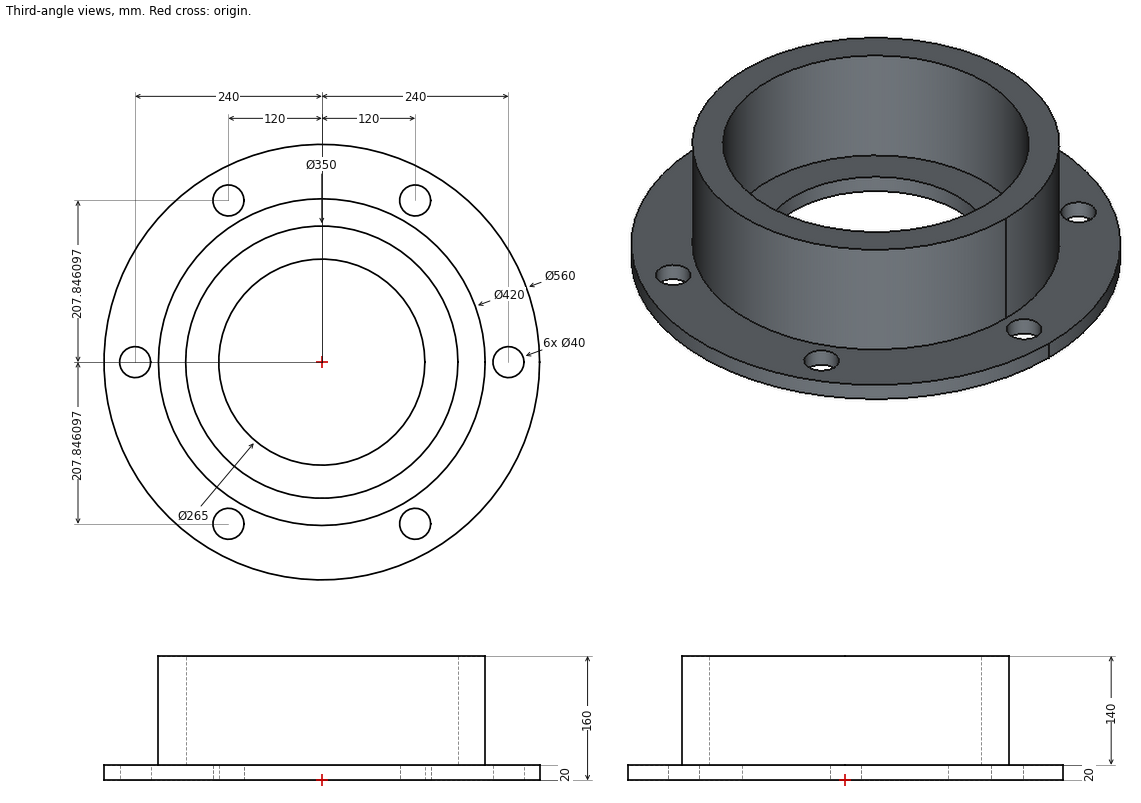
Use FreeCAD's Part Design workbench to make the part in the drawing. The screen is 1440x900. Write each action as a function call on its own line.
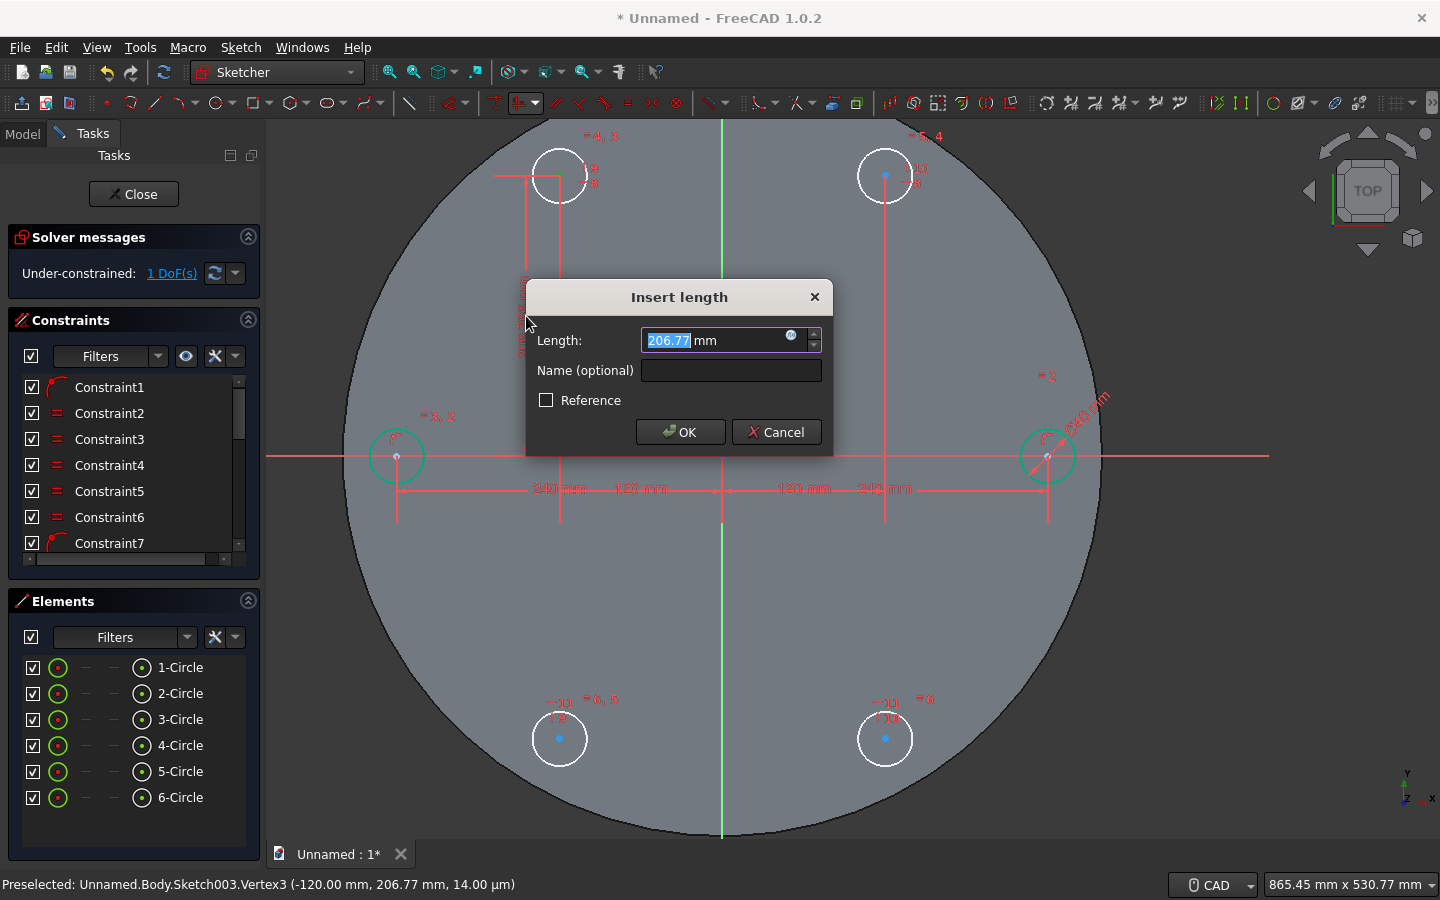
text(207.846097)
key(Return)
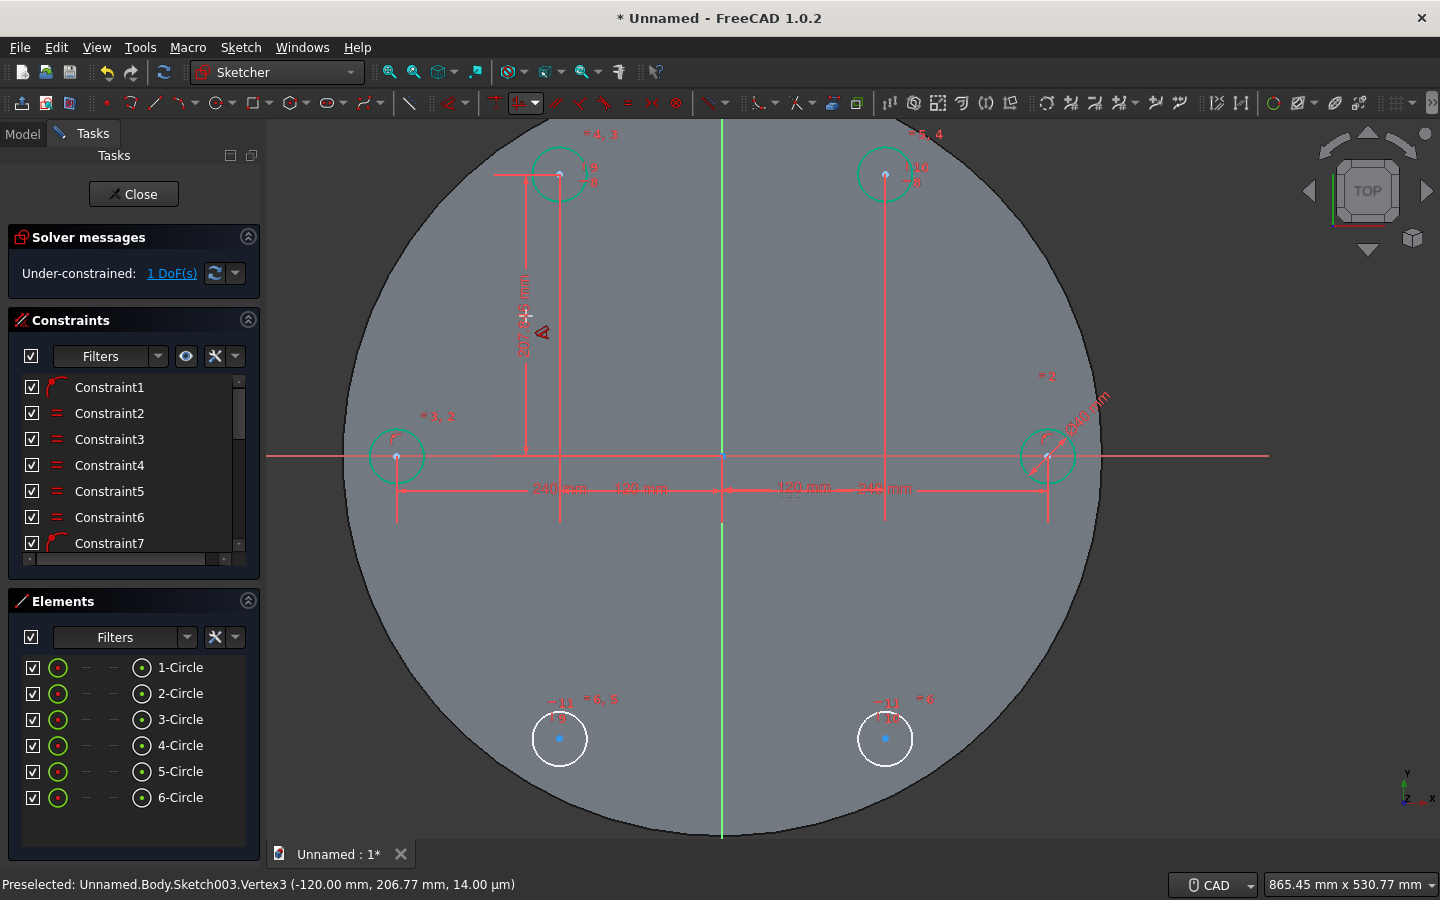
click(560, 739)
click(526, 598)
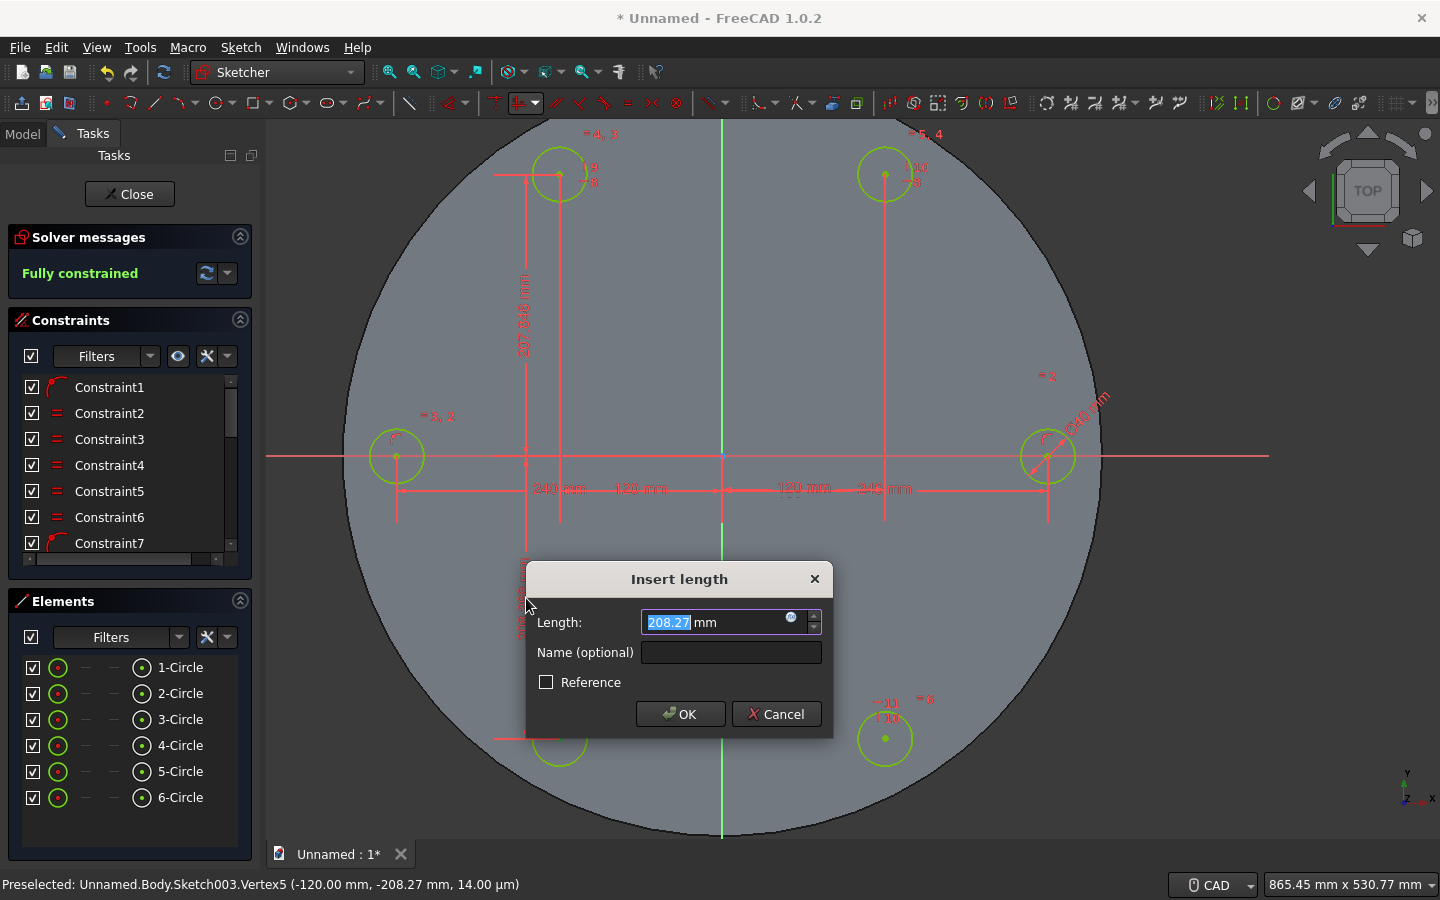
text(207.846097)
key(Return)
key(Escape)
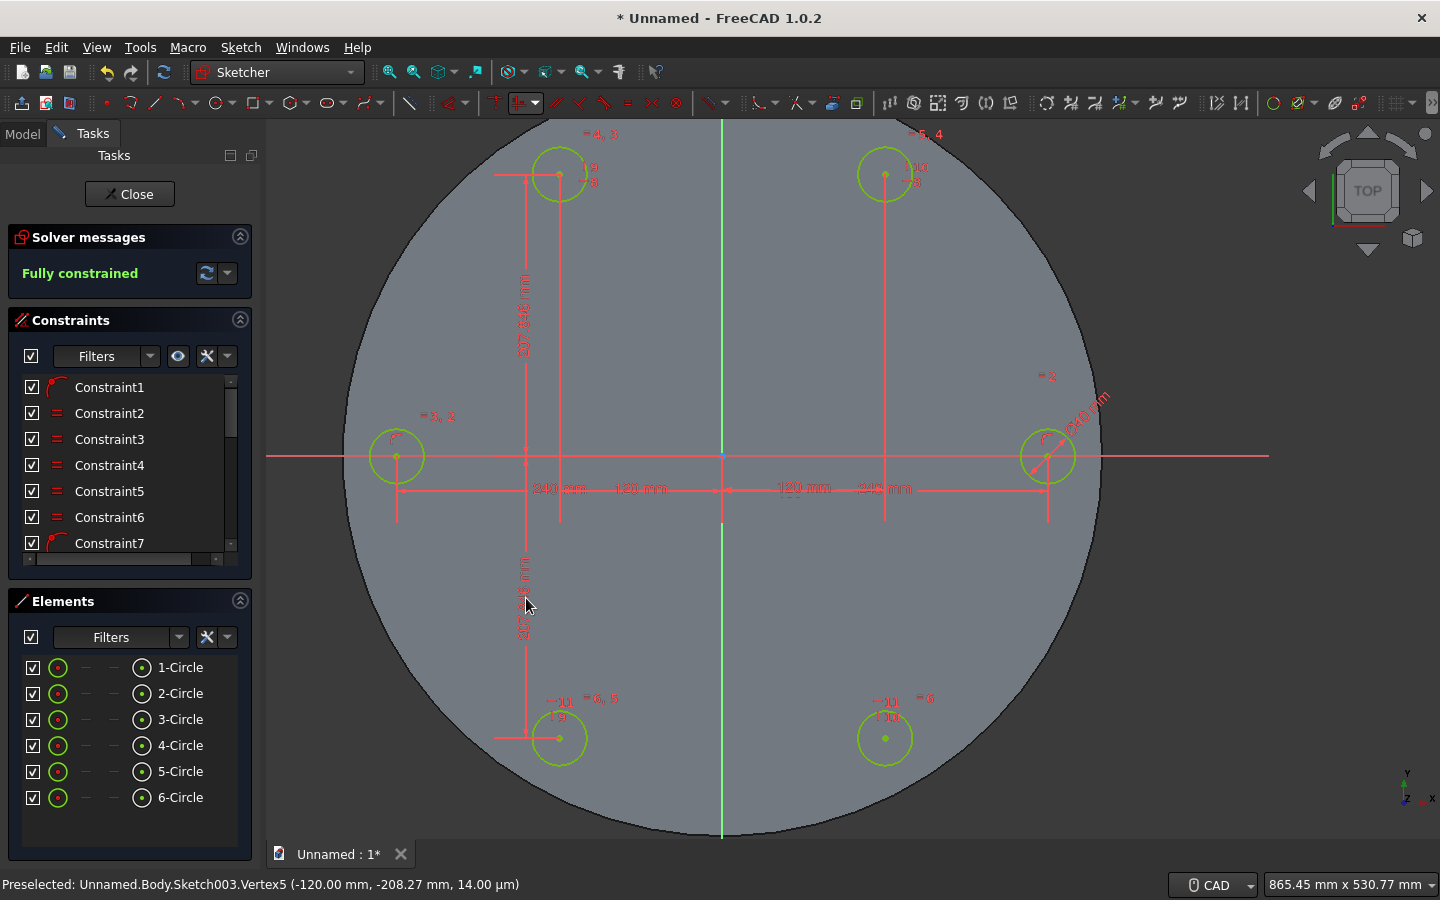
click(130, 194)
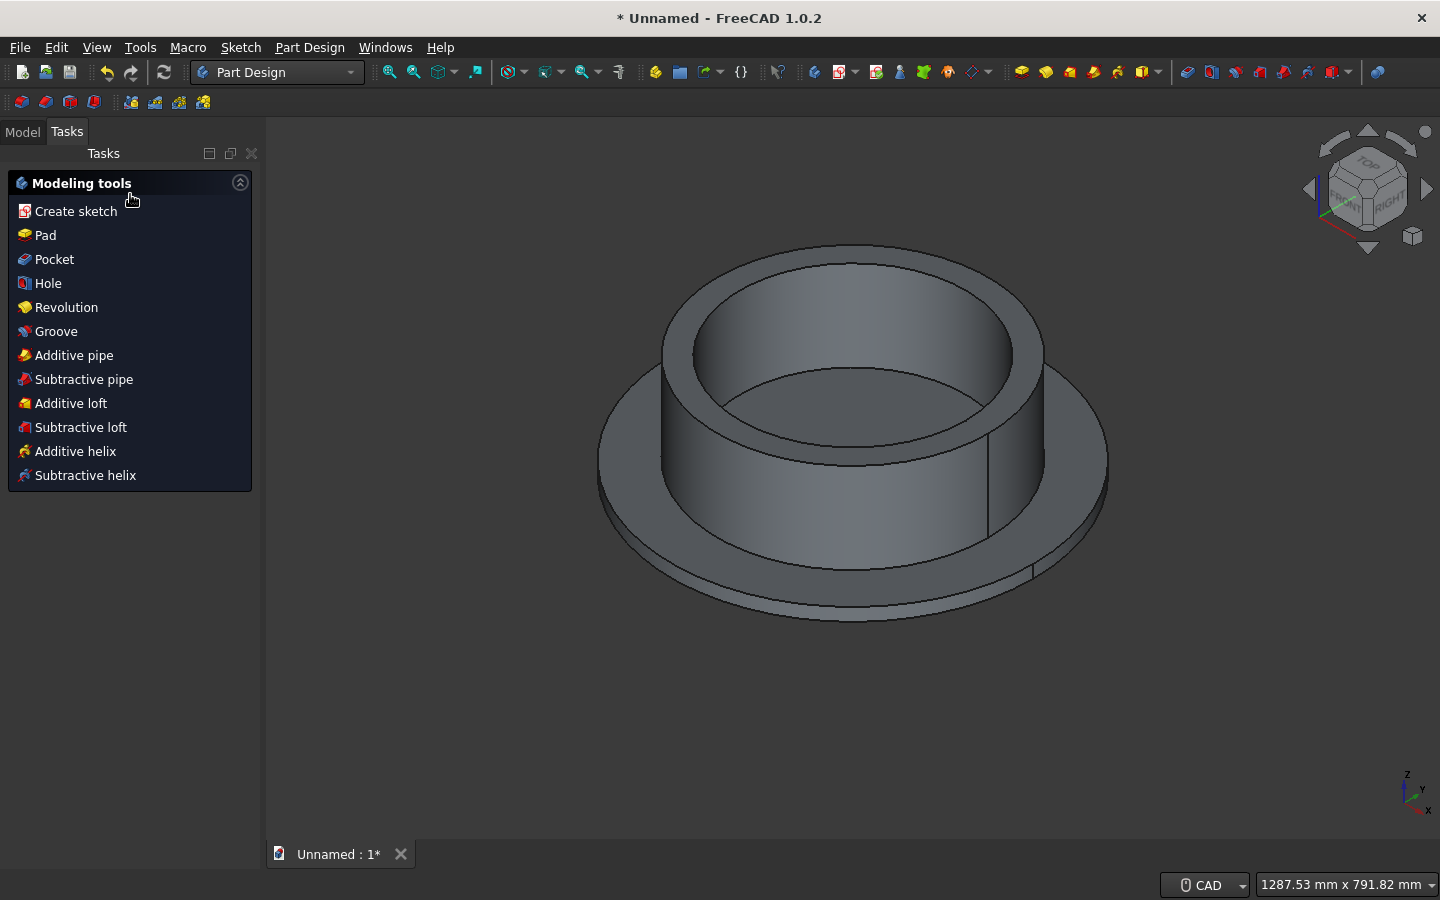
click(1188, 72)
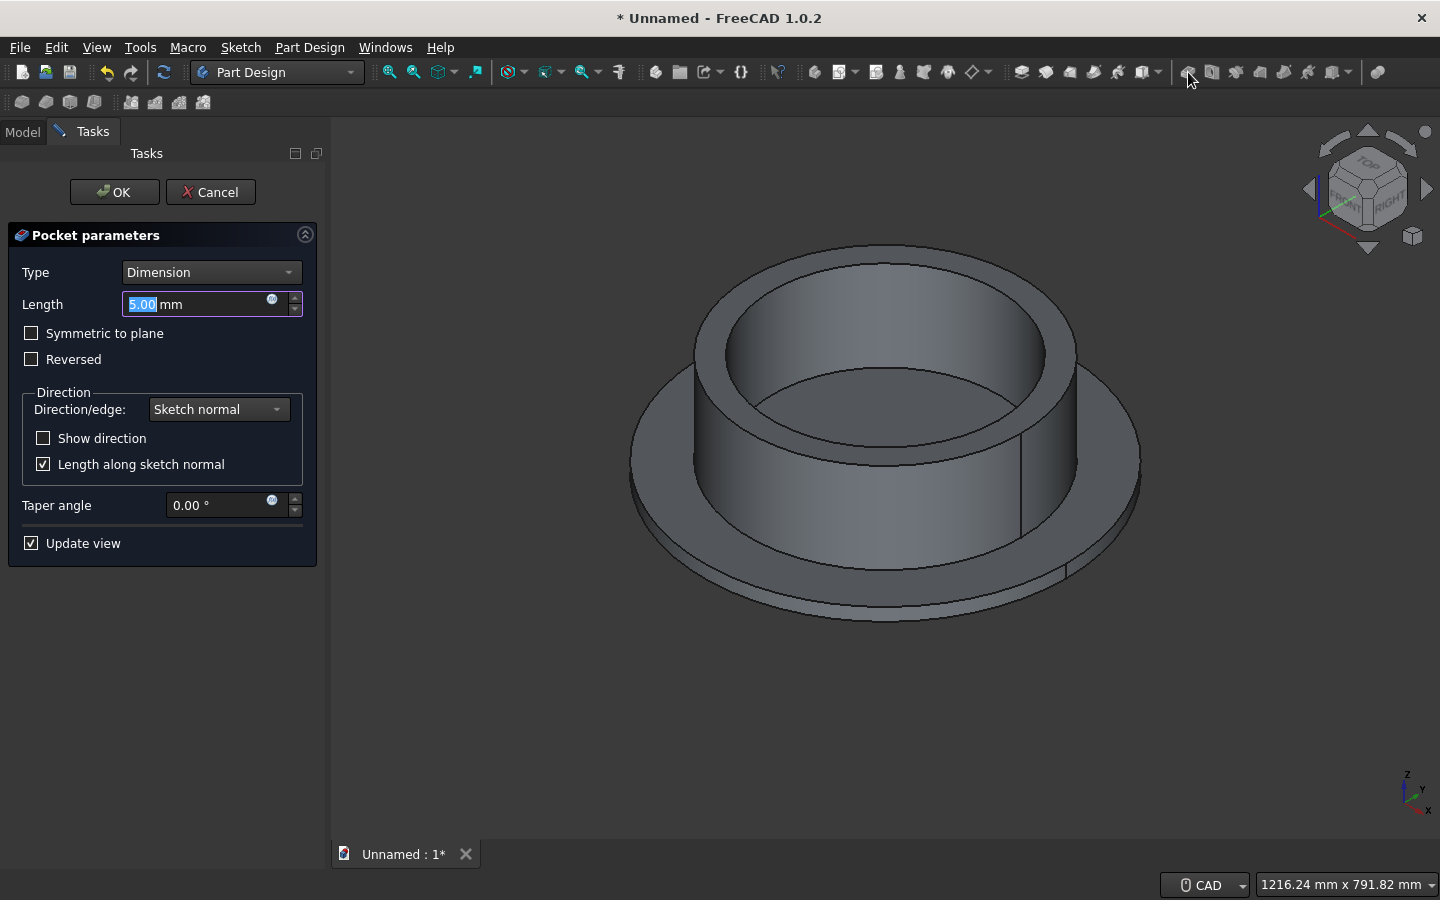
text(20)
key(Tab)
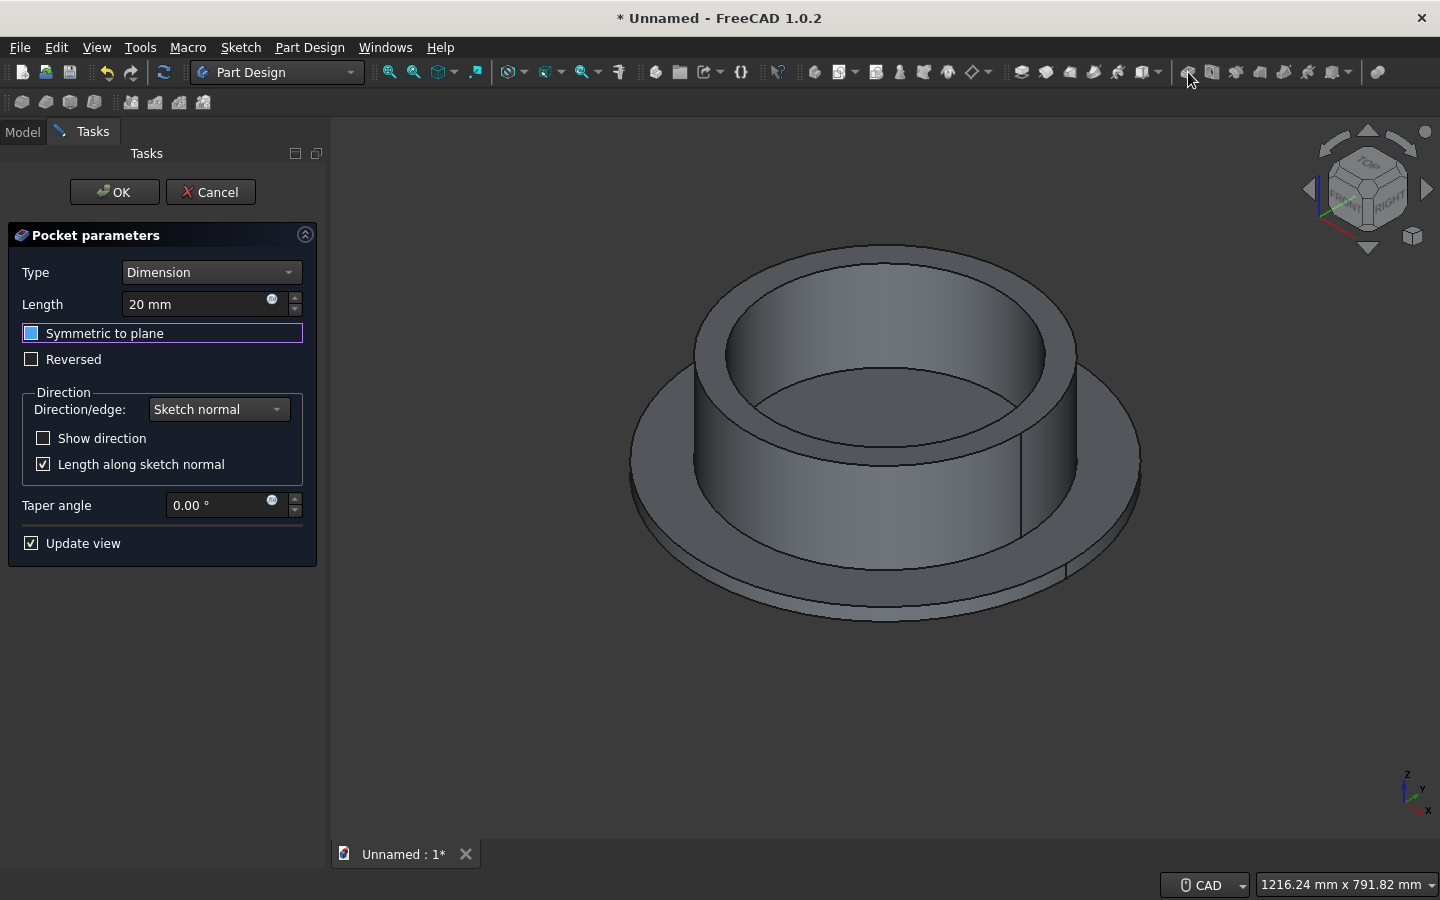
click(30, 359)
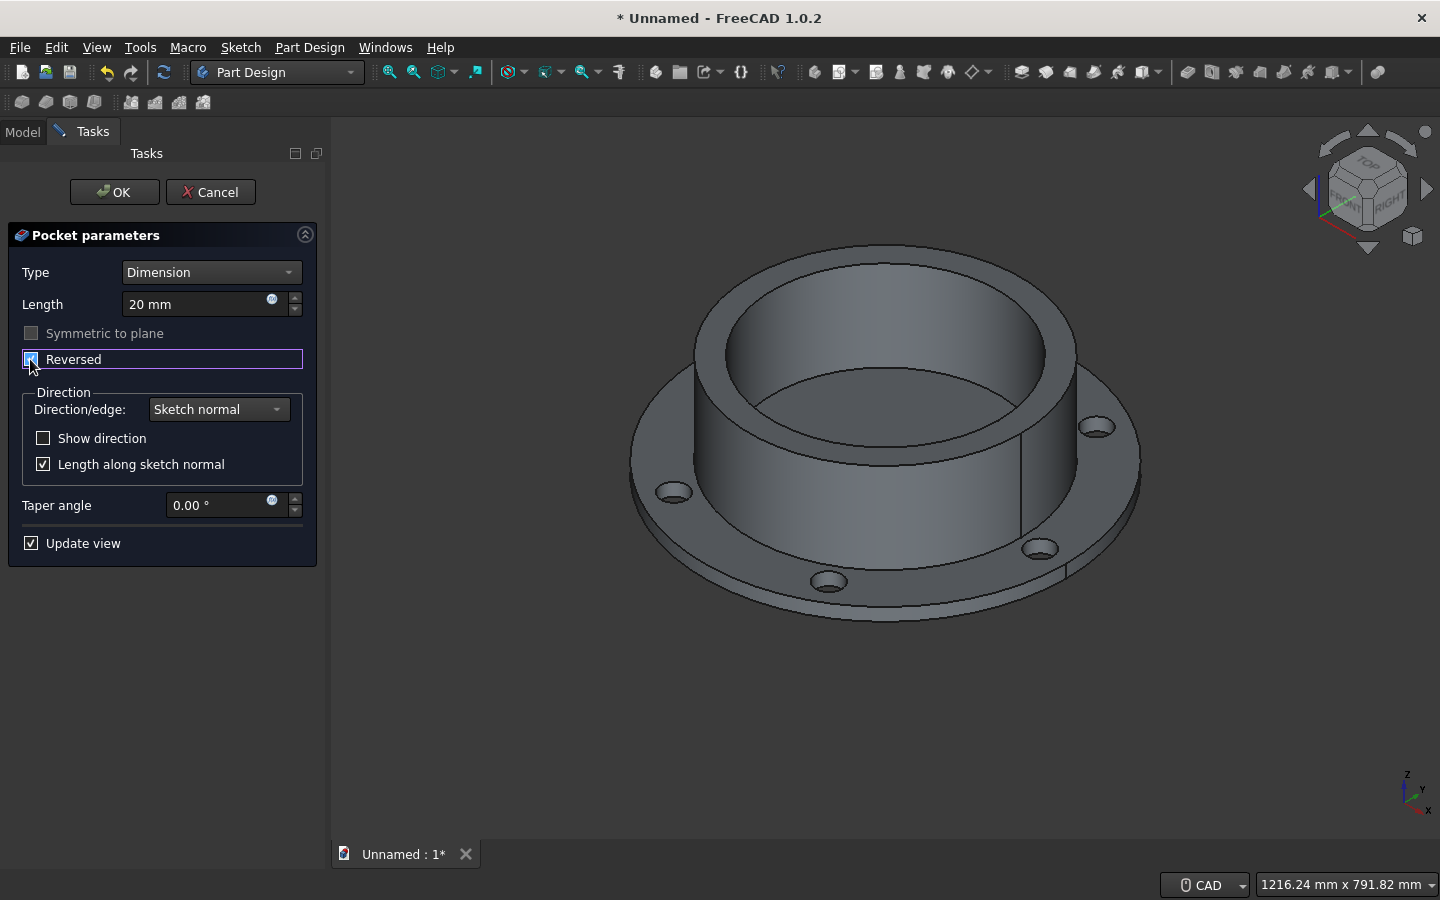
click(115, 192)